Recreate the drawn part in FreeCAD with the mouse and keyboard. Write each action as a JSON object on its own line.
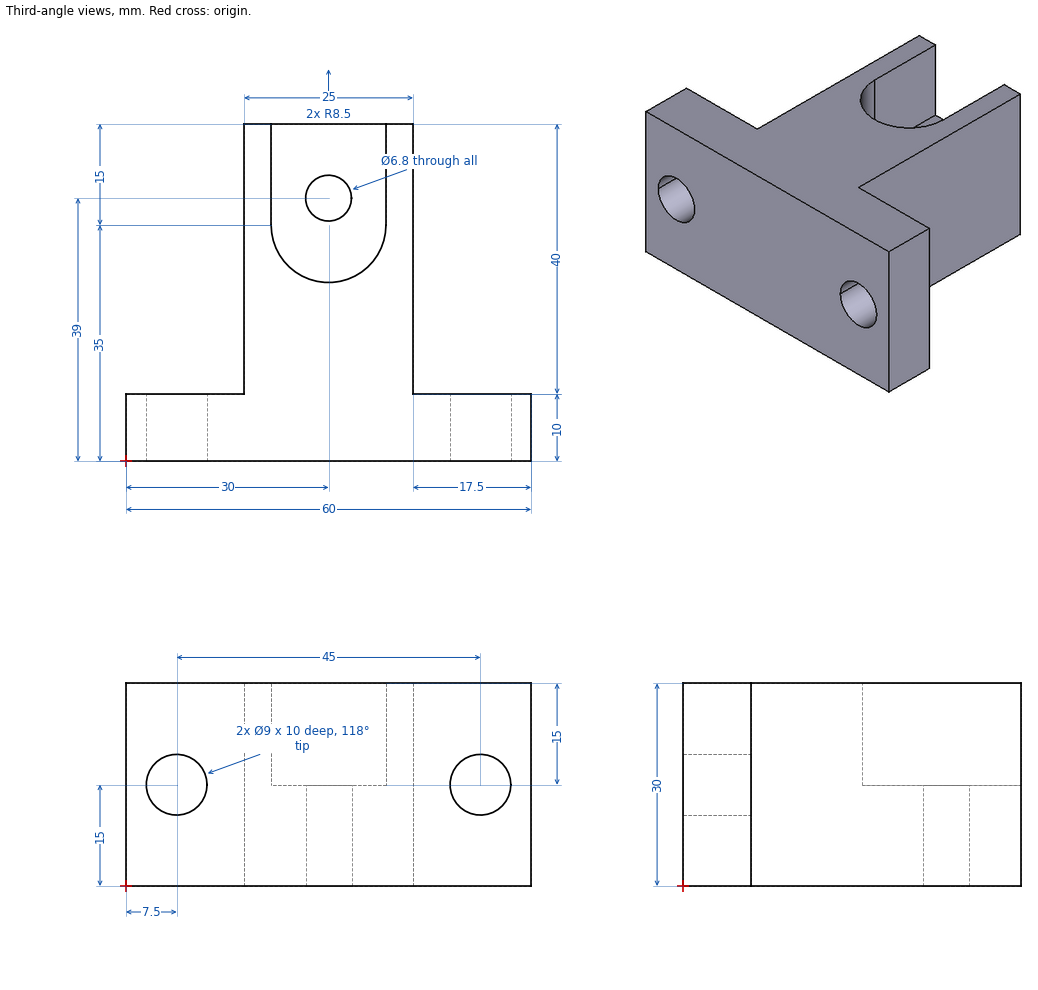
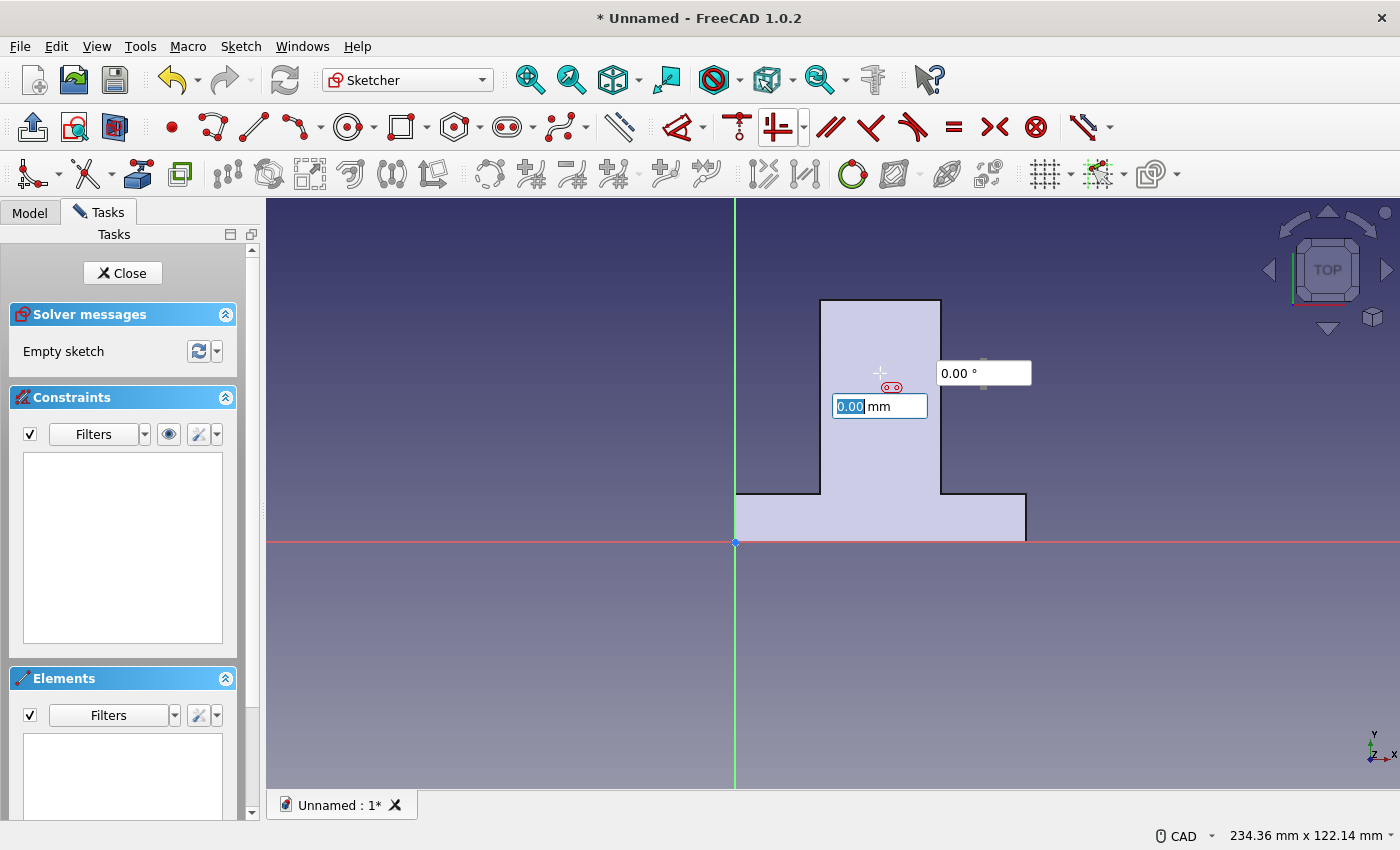
{"action": "left_click", "coordinate": [880, 300]}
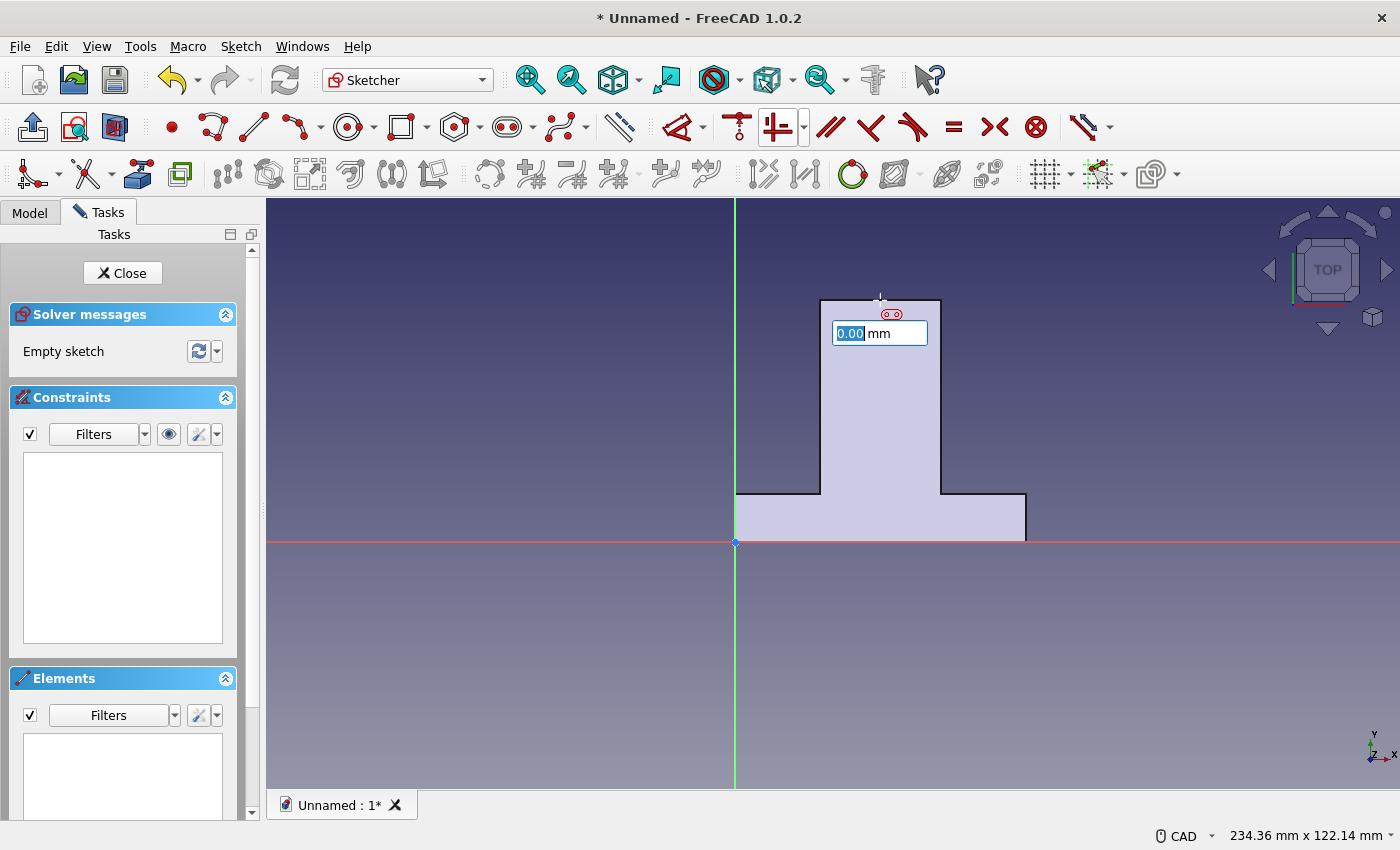
{"action": "left_click", "coordinate": [922, 337]}
{"action": "key", "text": "Escape"}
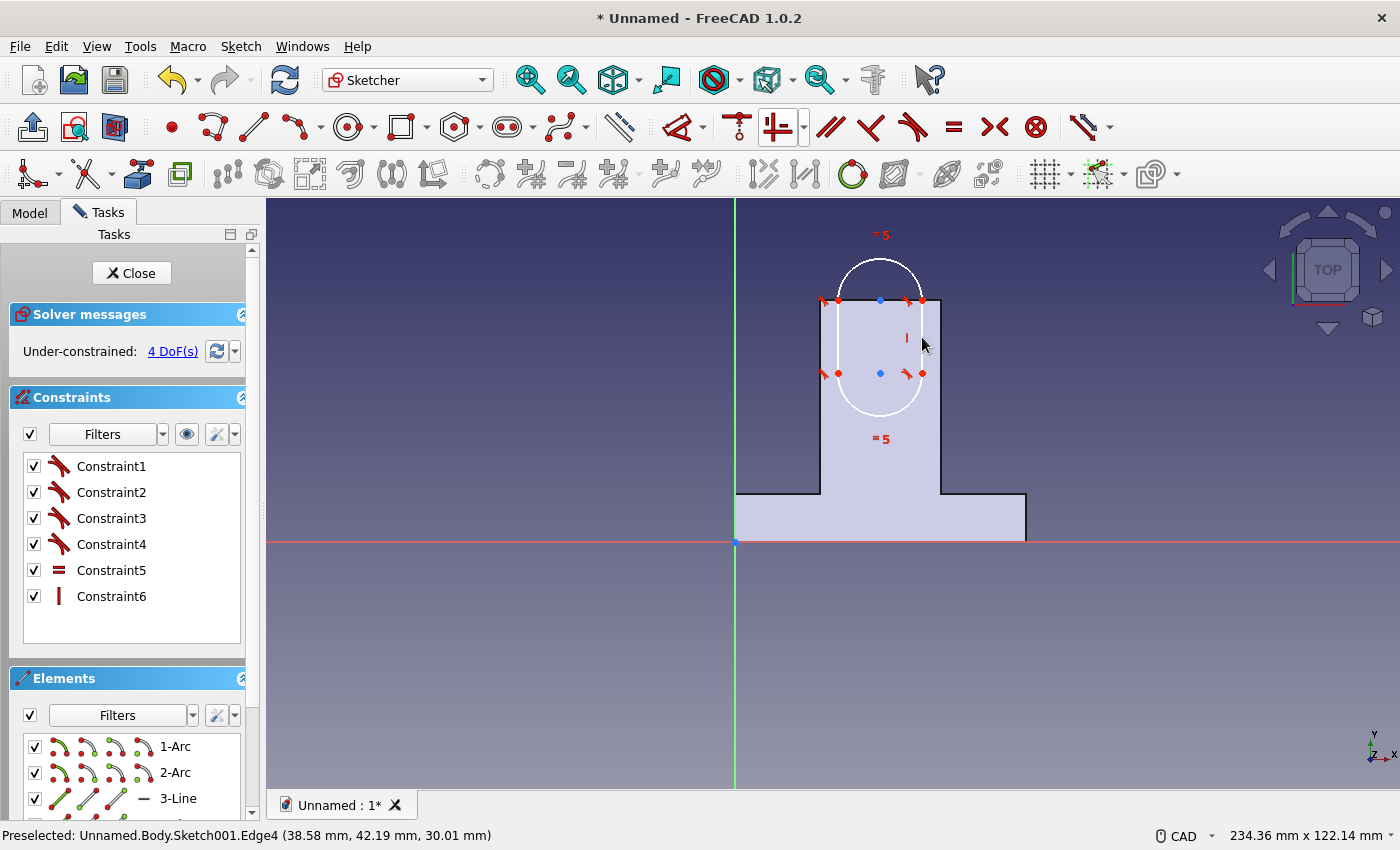
{"action": "left_click", "coordinate": [676, 128]}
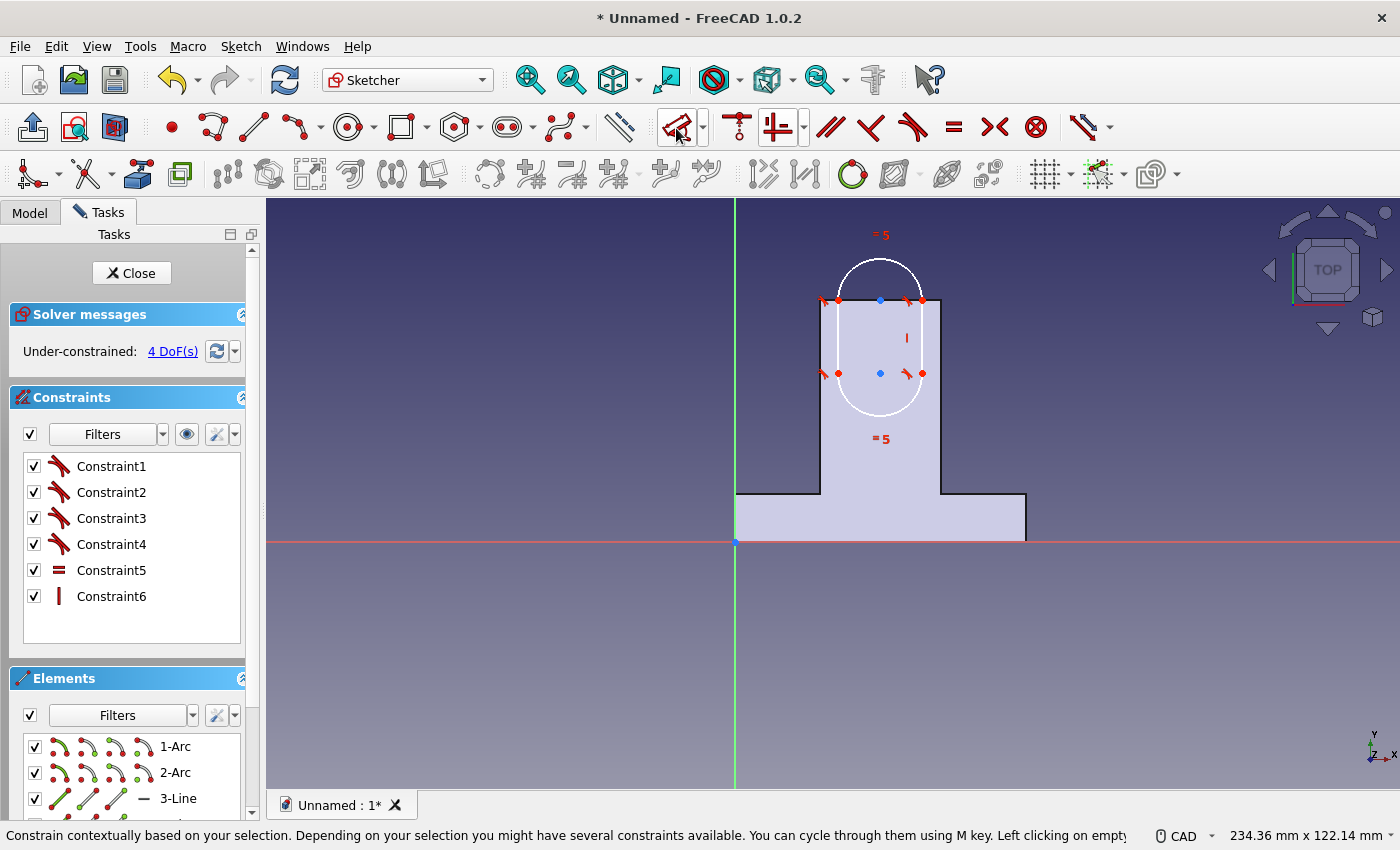
{"action": "left_click", "coordinate": [855, 408]}
{"action": "left_click", "coordinate": [836, 434]}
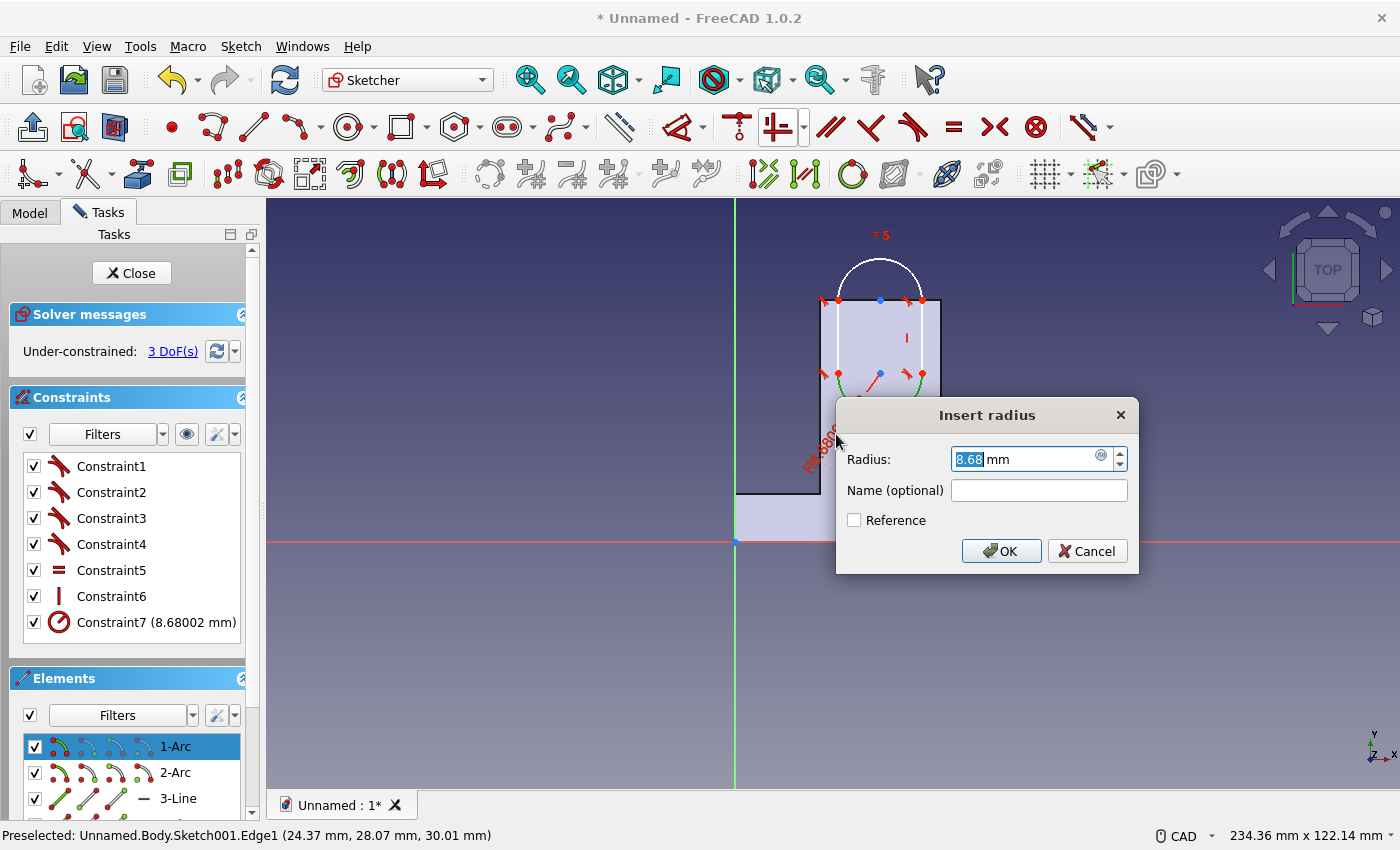
{"action": "type", "text": "8.5"}
{"action": "key", "text": "Return"}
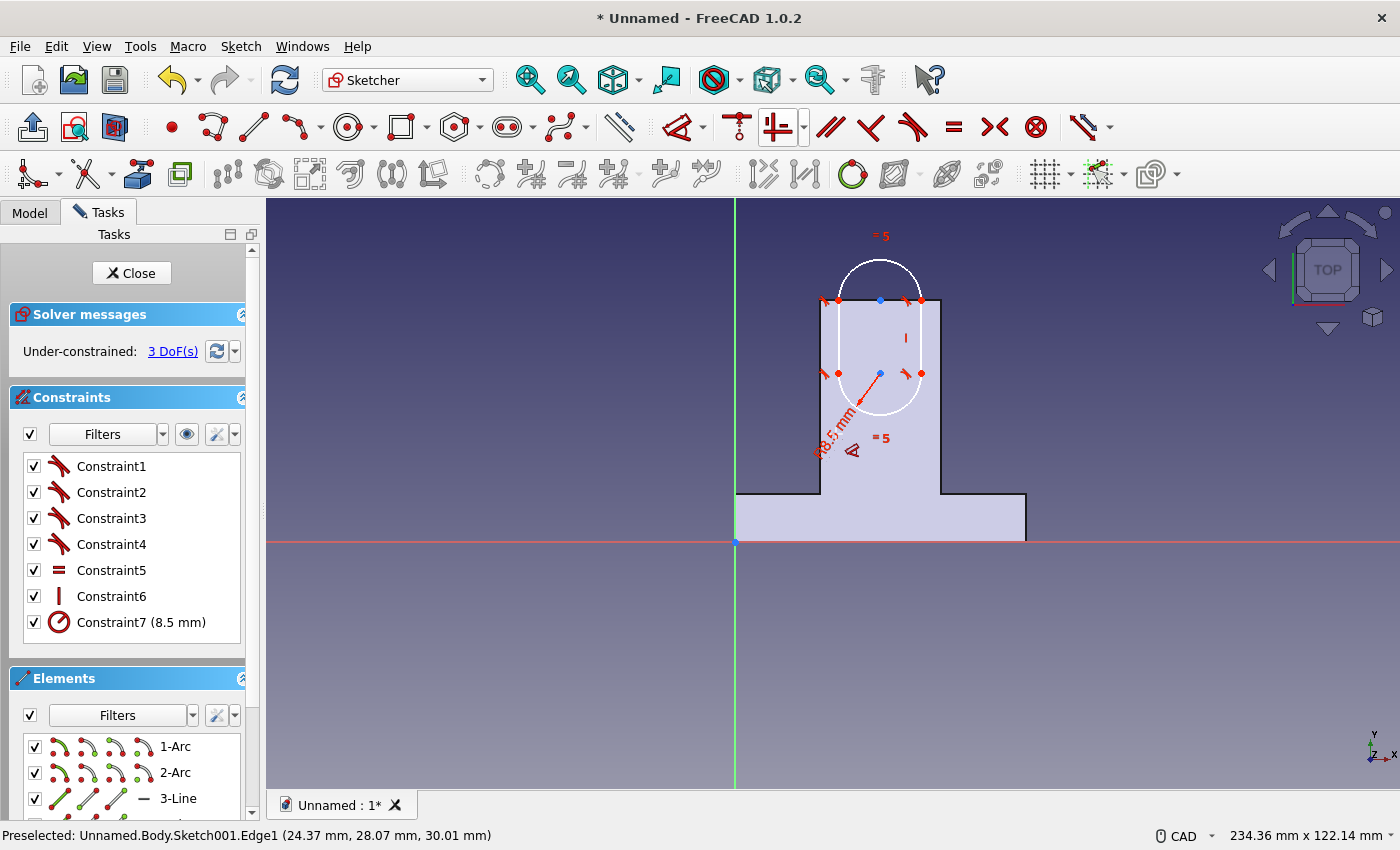
{"action": "left_click", "coordinate": [839, 352]}
{"action": "left_click", "coordinate": [873, 338]}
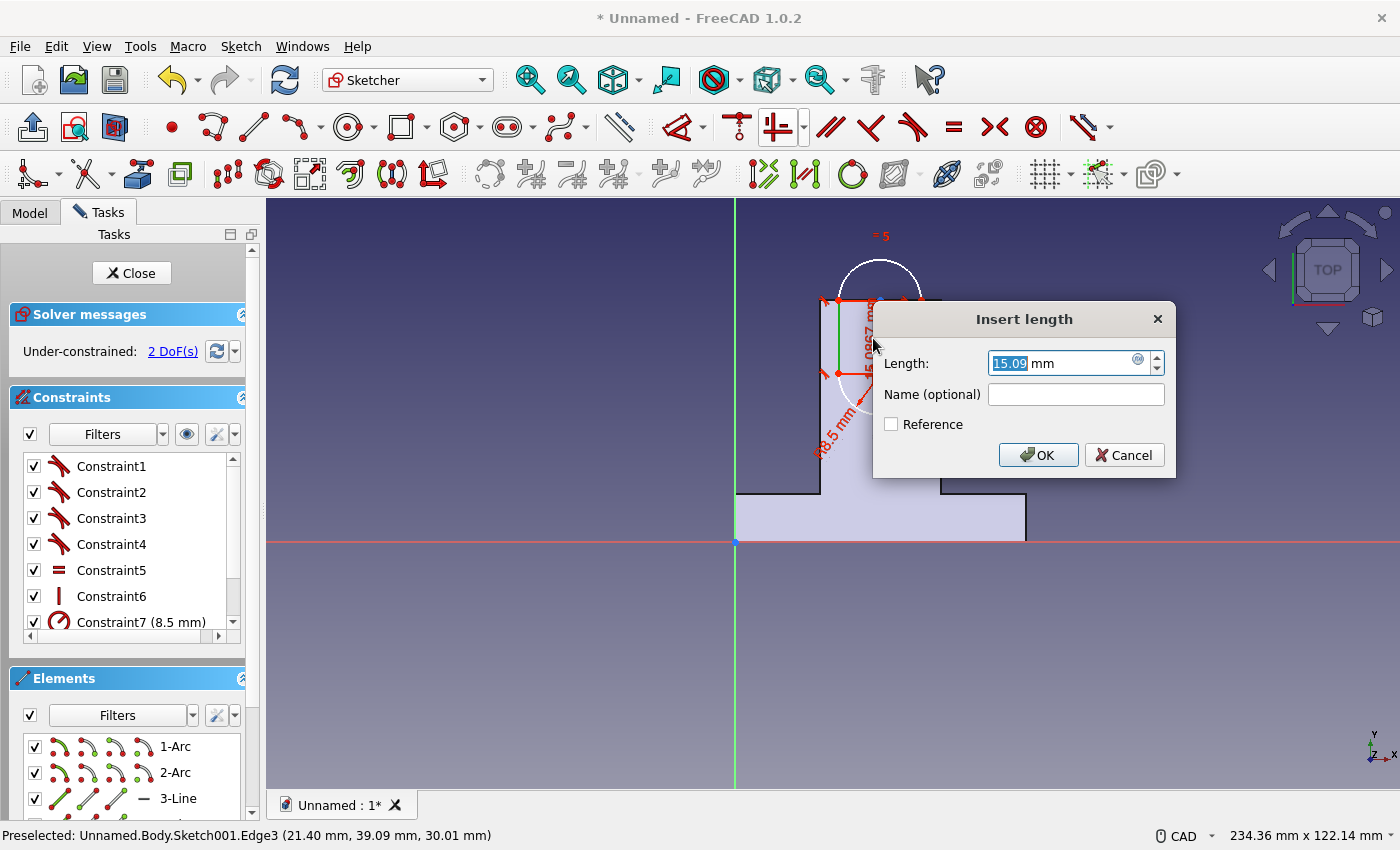
{"action": "type", "text": "15"}
{"action": "key", "text": "Return"}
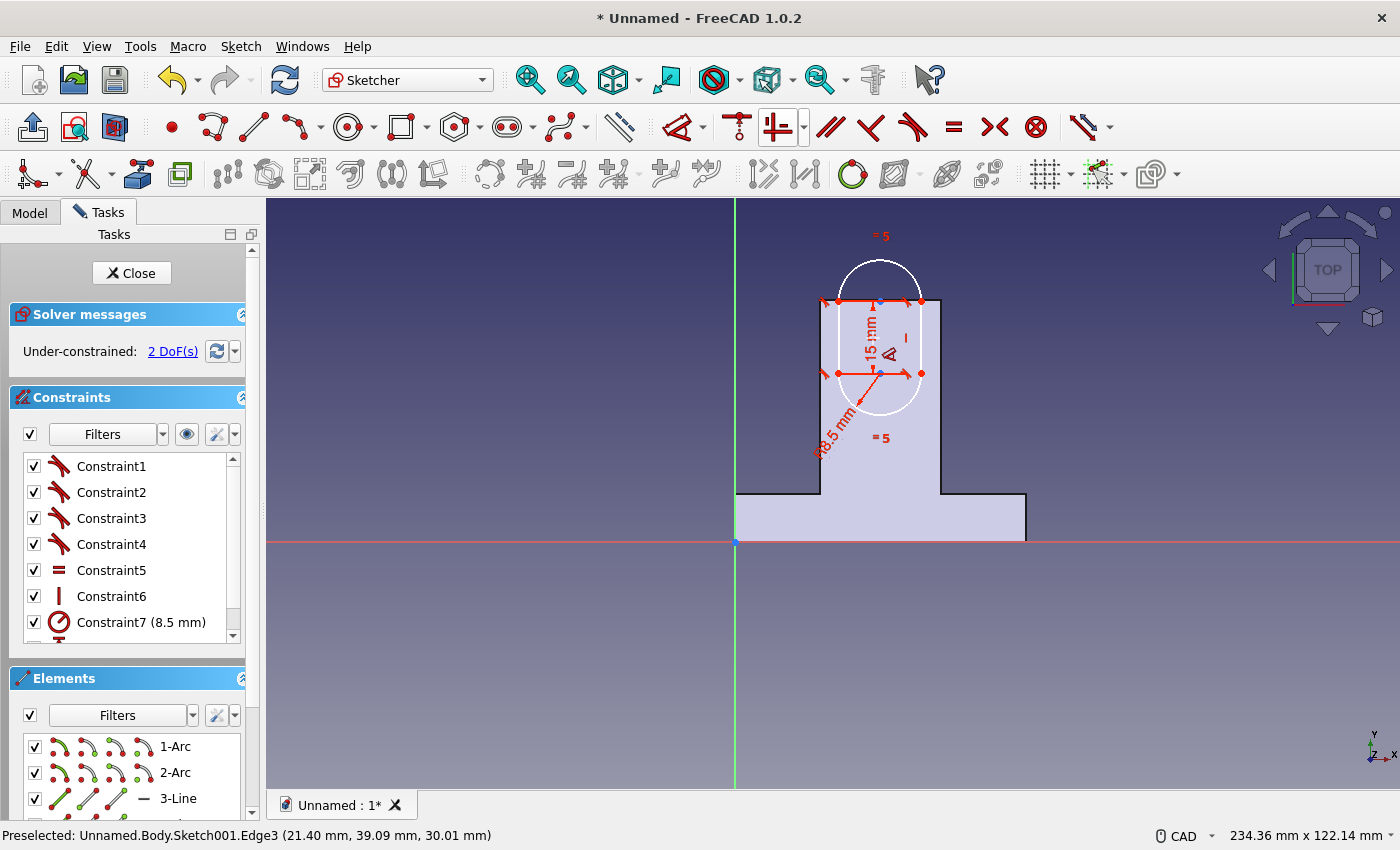
{"action": "left_click", "coordinate": [839, 374]}
{"action": "left_click", "coordinate": [701, 458]}